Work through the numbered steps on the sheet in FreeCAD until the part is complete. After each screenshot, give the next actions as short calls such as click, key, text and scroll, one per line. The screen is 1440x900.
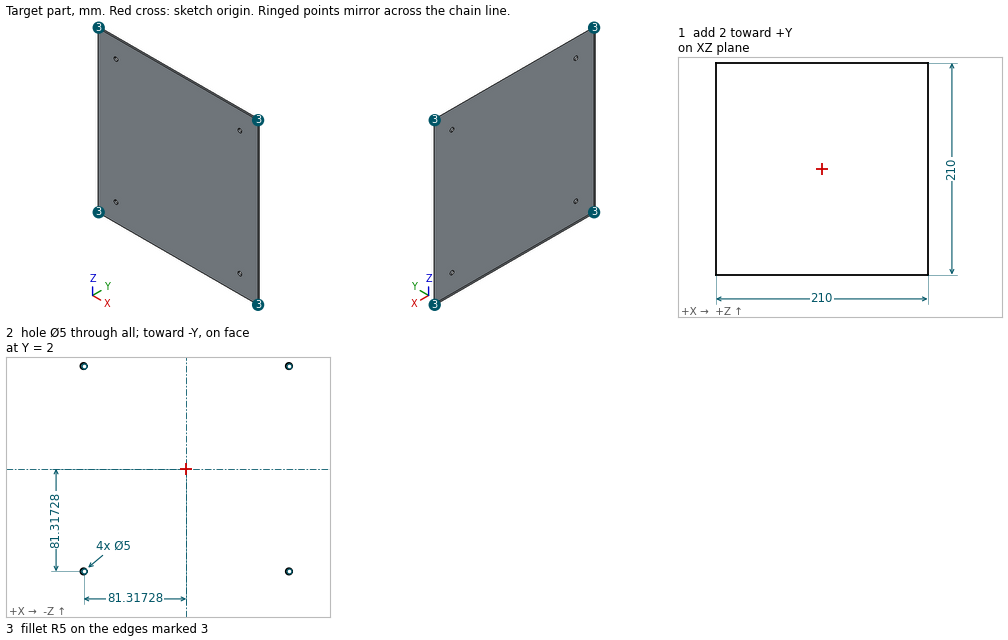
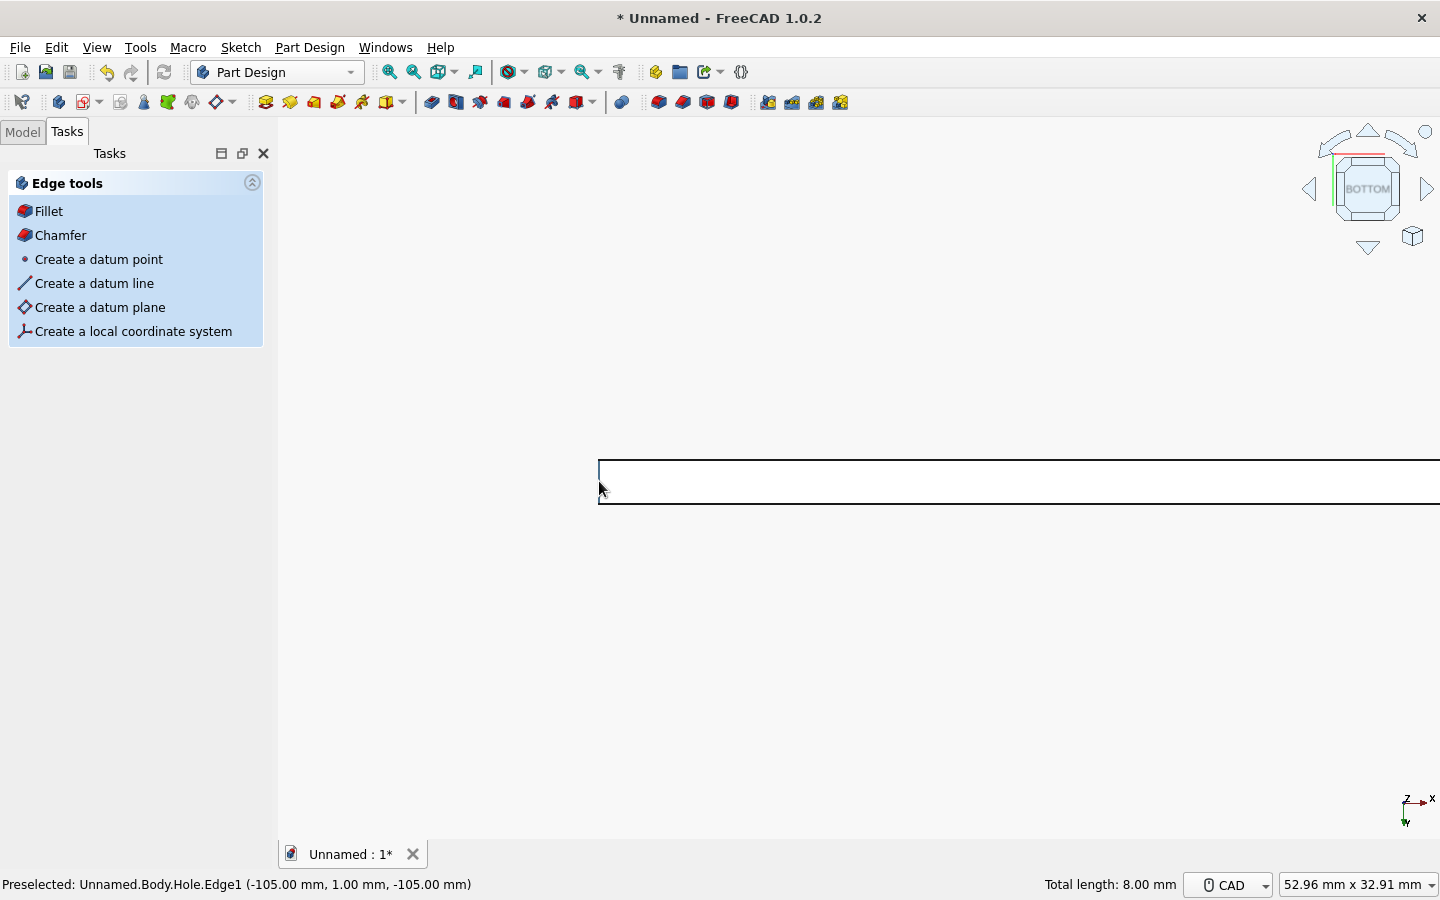
click(660, 102)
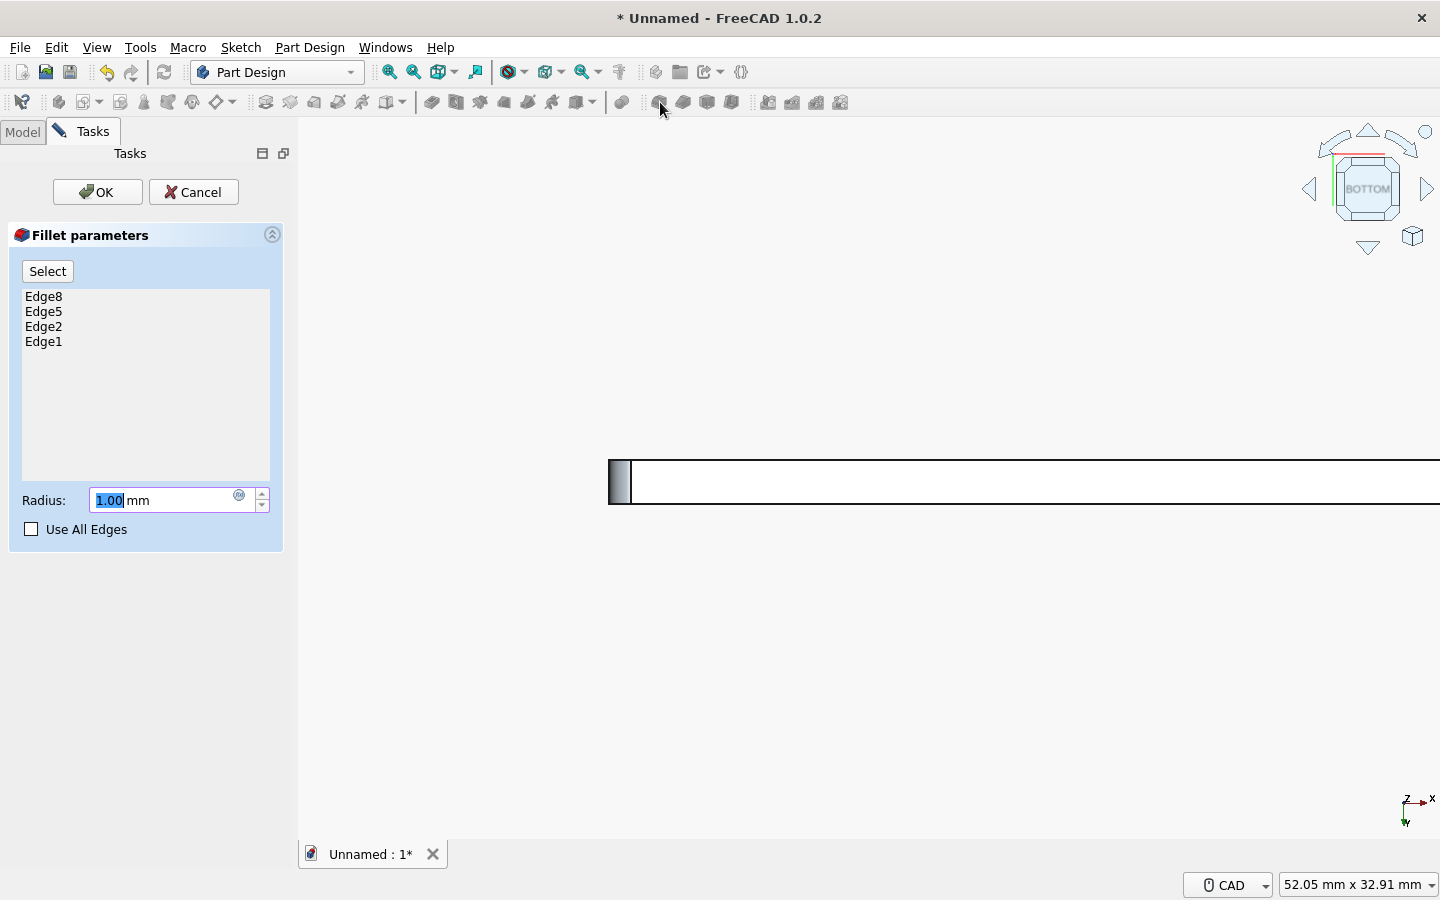
text(5)
key(Tab)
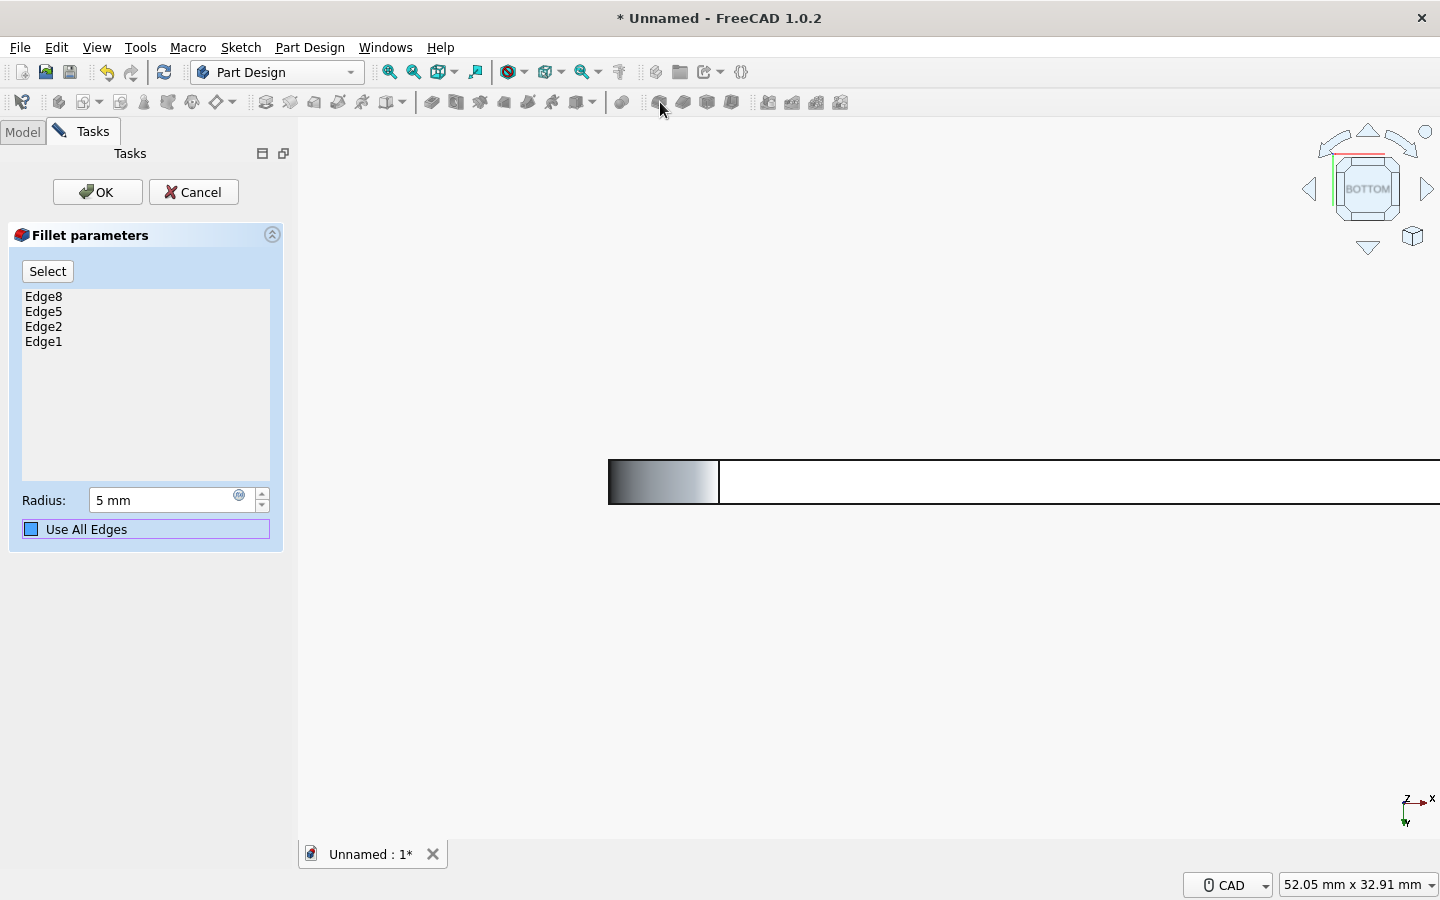
click(98, 192)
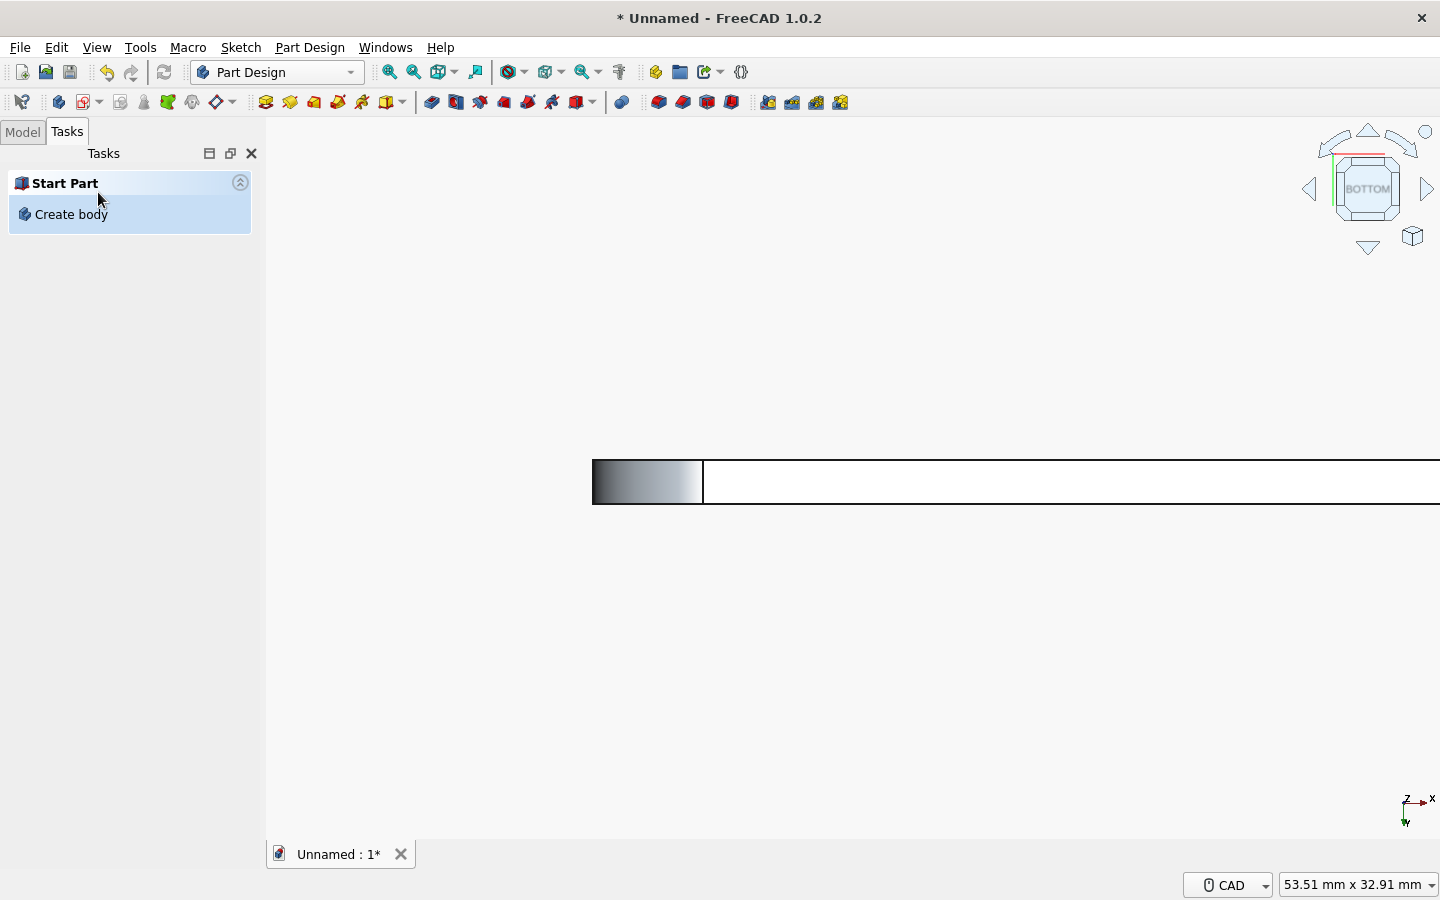
key(0)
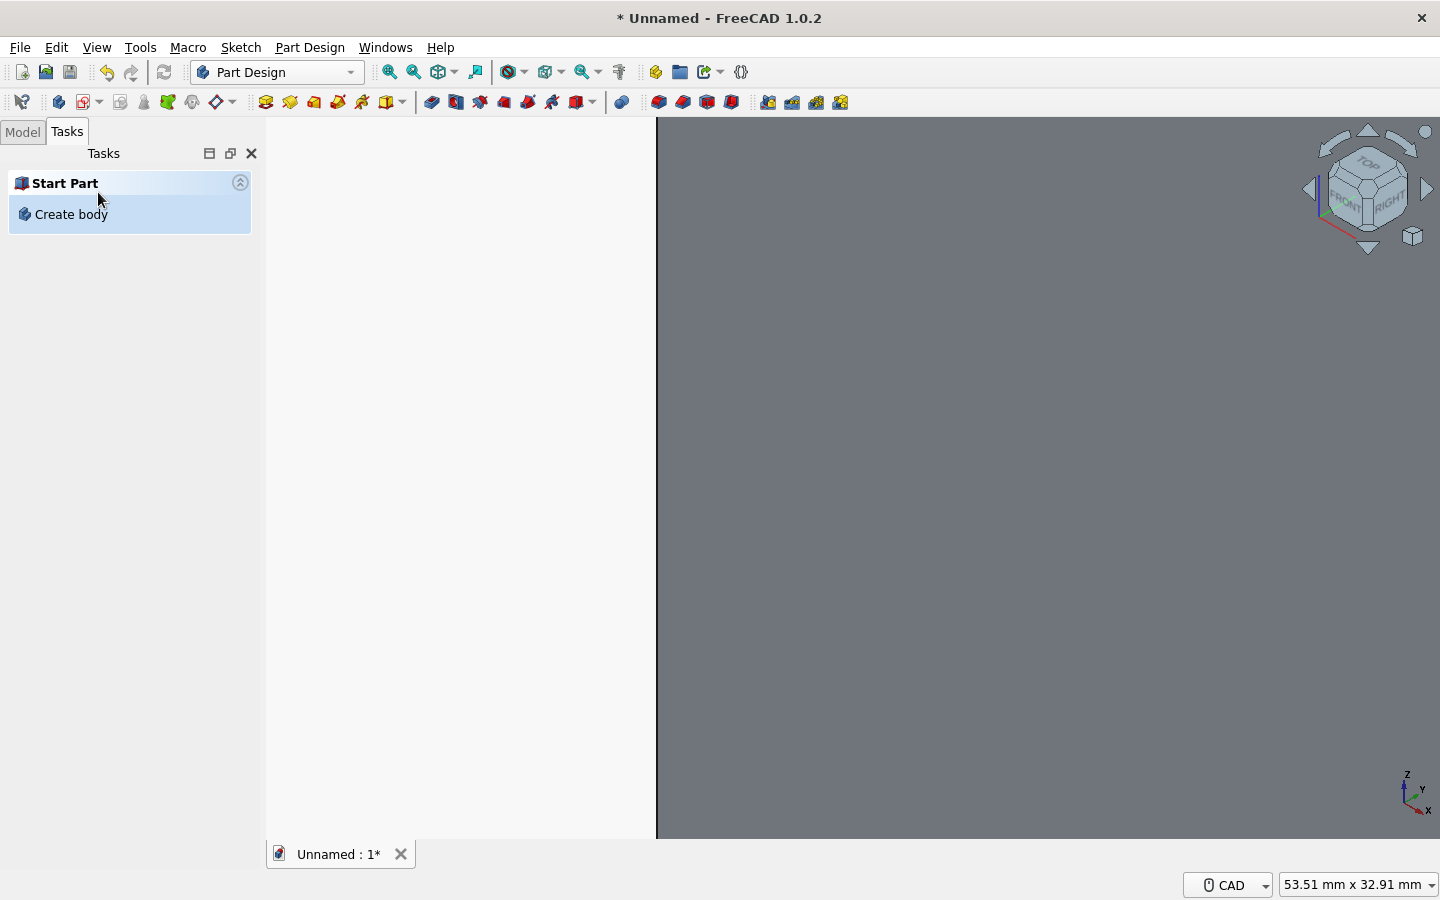
click(390, 72)